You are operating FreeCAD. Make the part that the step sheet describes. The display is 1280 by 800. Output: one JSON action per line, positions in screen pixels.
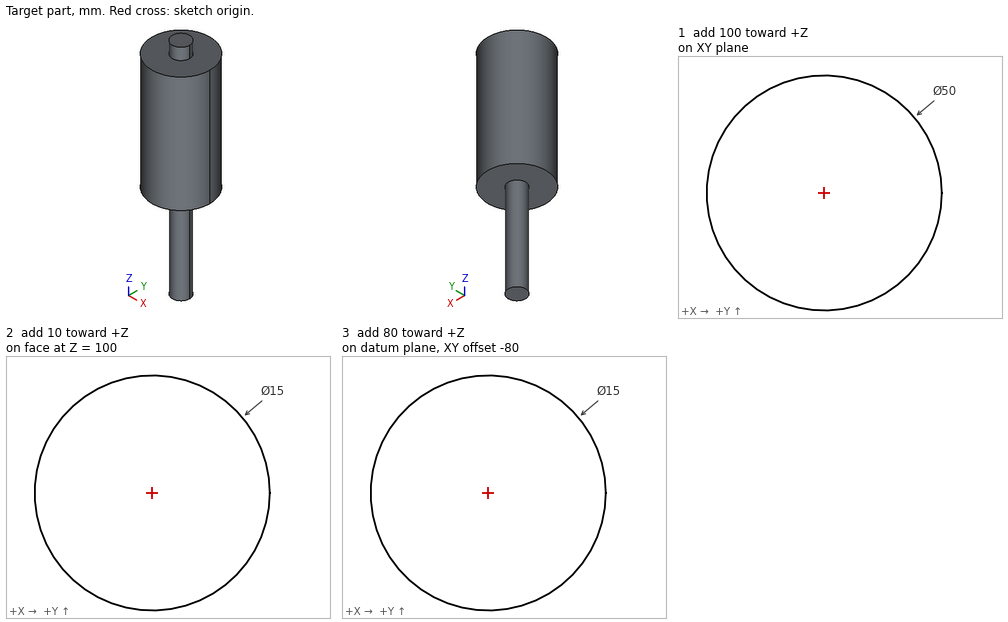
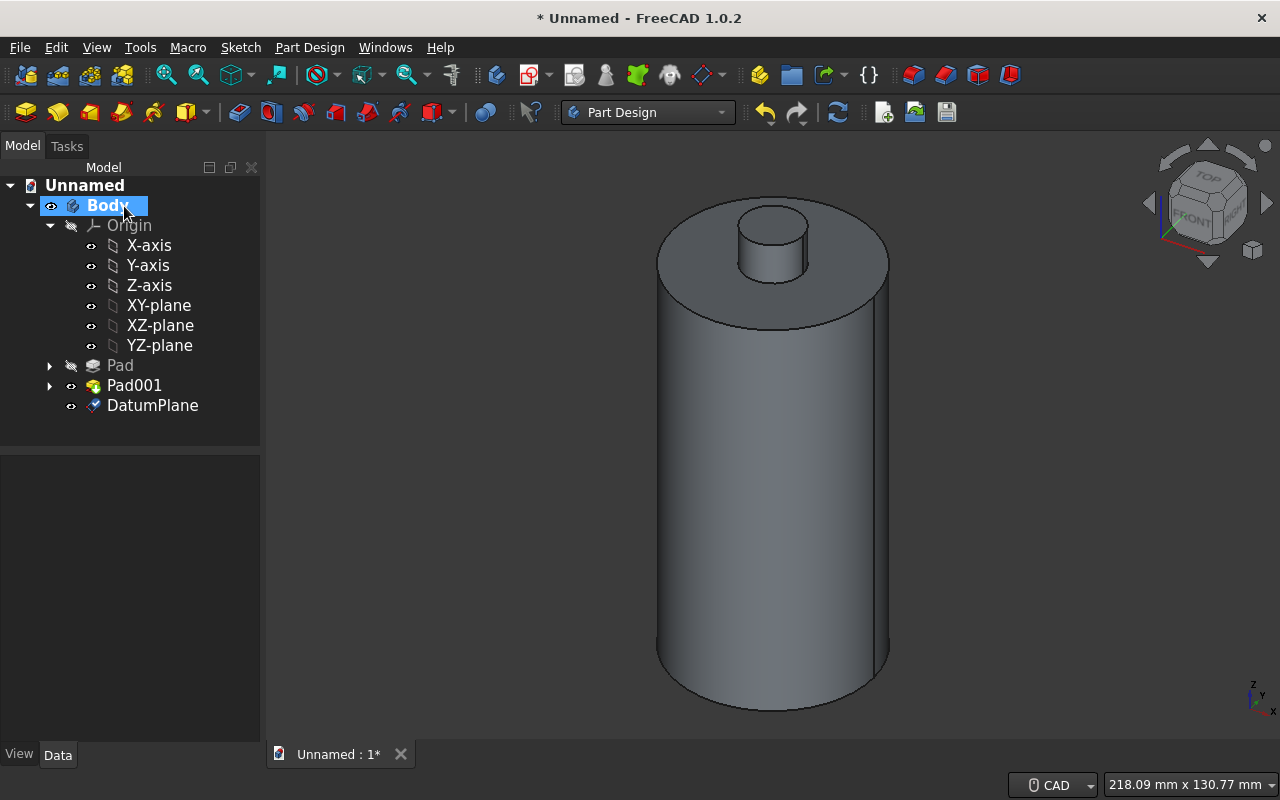
{"action": "left_click", "coordinate": [116, 406]}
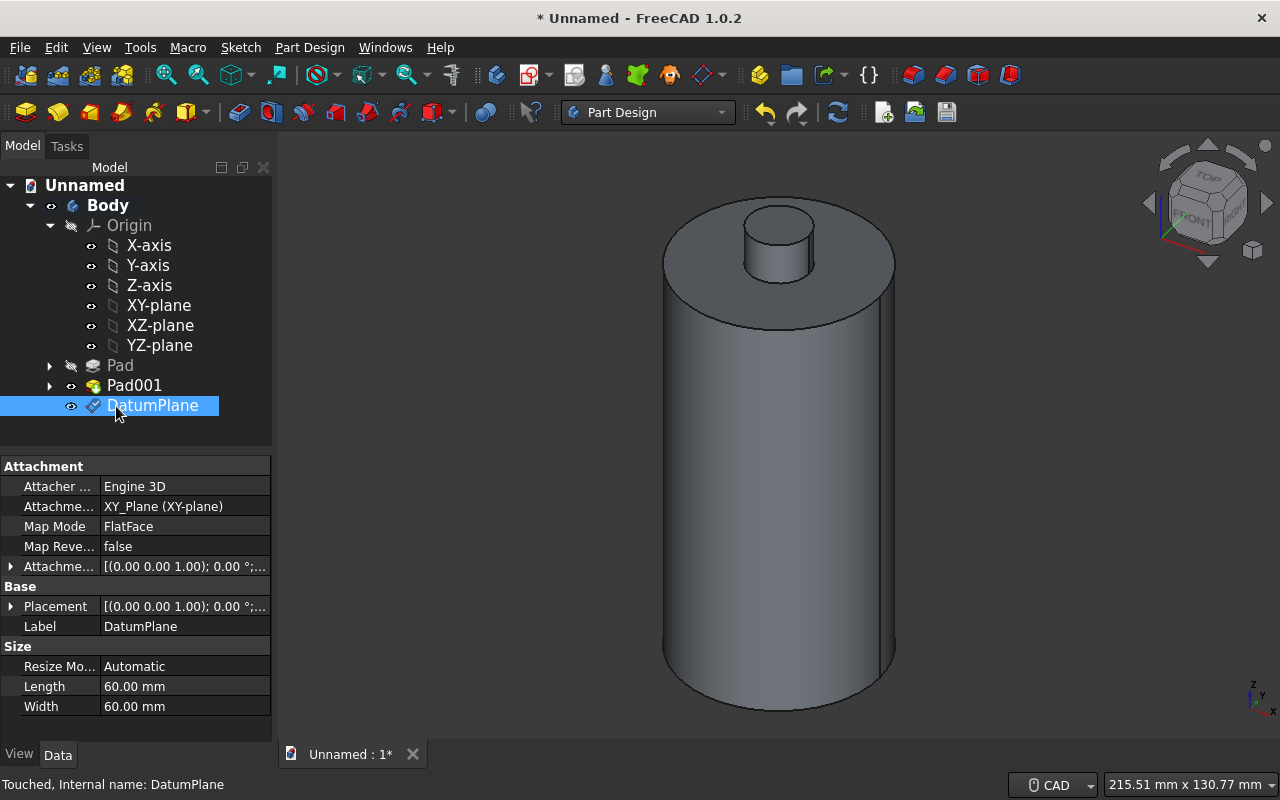
{"action": "left_click", "coordinate": [530, 76]}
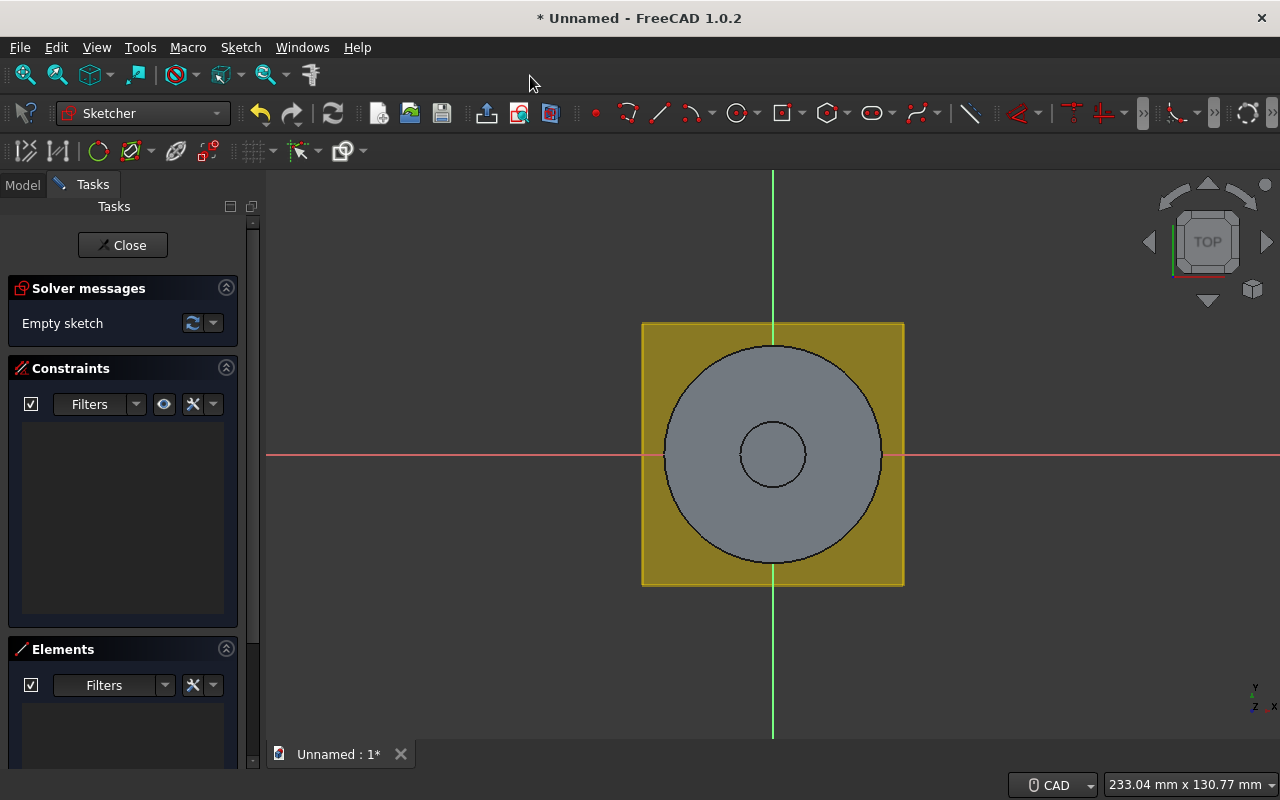
{"action": "left_click", "coordinate": [552, 114]}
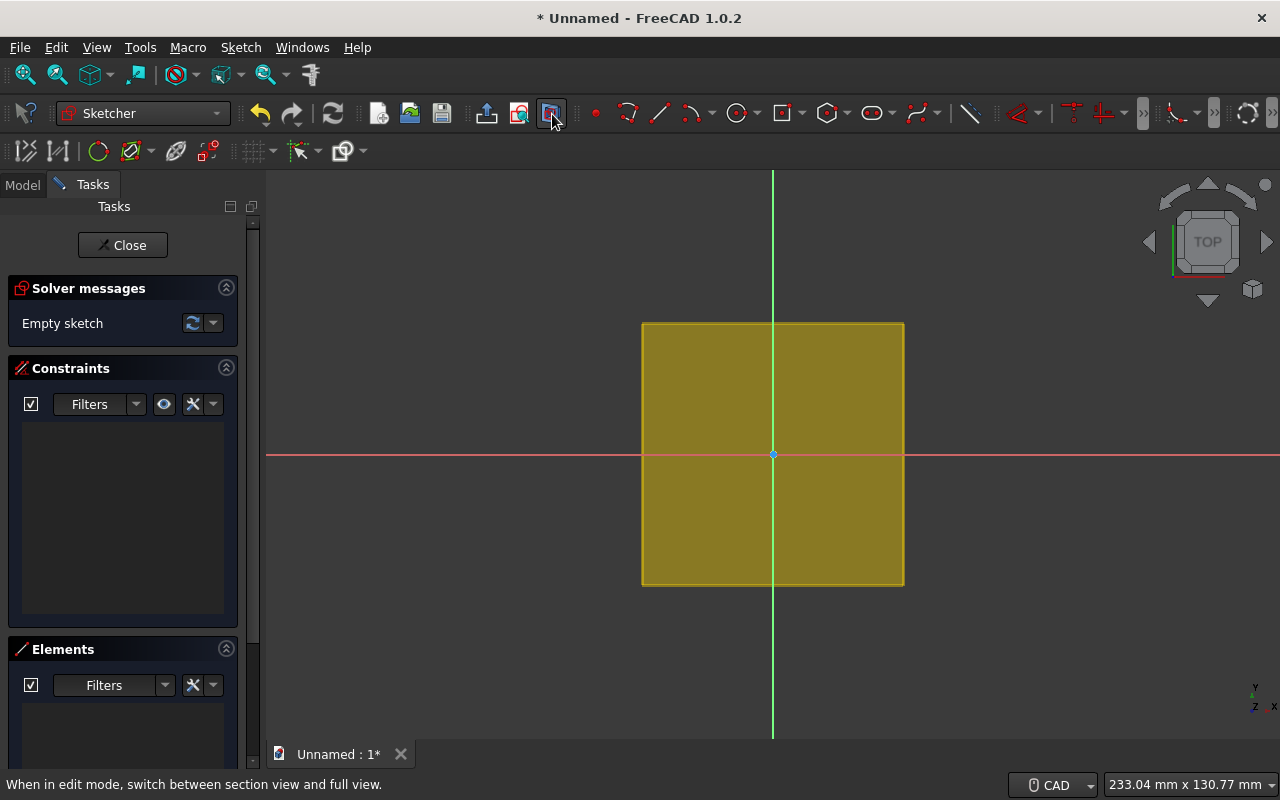
{"action": "scroll", "coordinate": [787, 455], "scroll_direction": "up", "scroll_amount": 9}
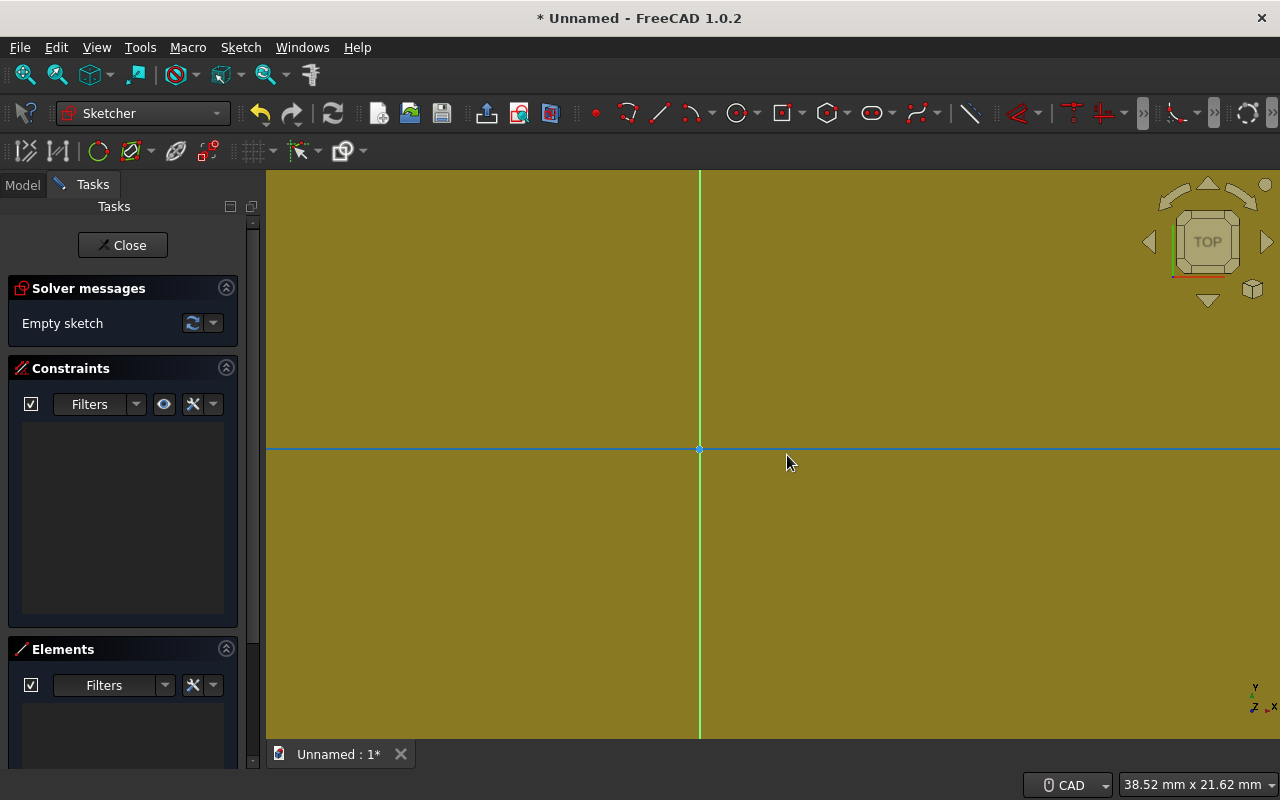
{"action": "left_click", "coordinate": [738, 114]}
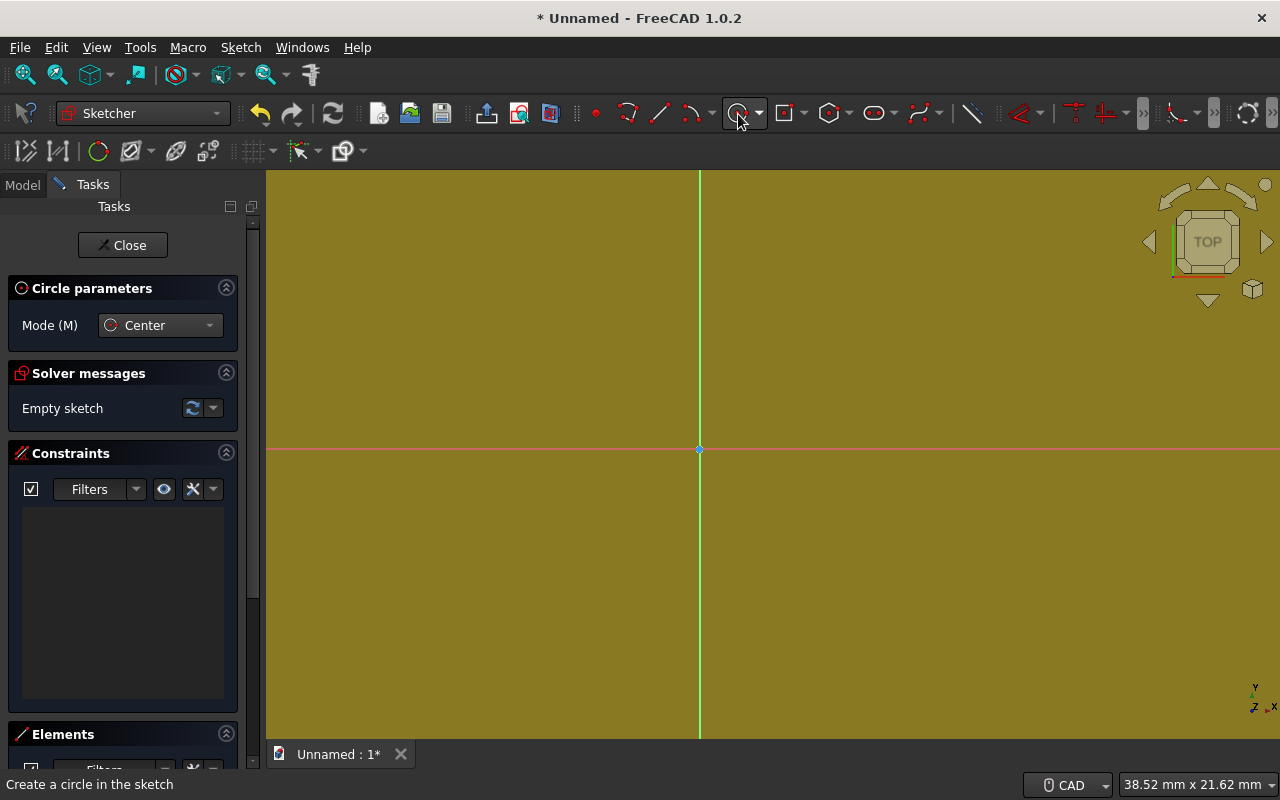
{"action": "left_click", "coordinate": [700, 449]}
{"action": "mouse_move", "coordinate": [839, 310]}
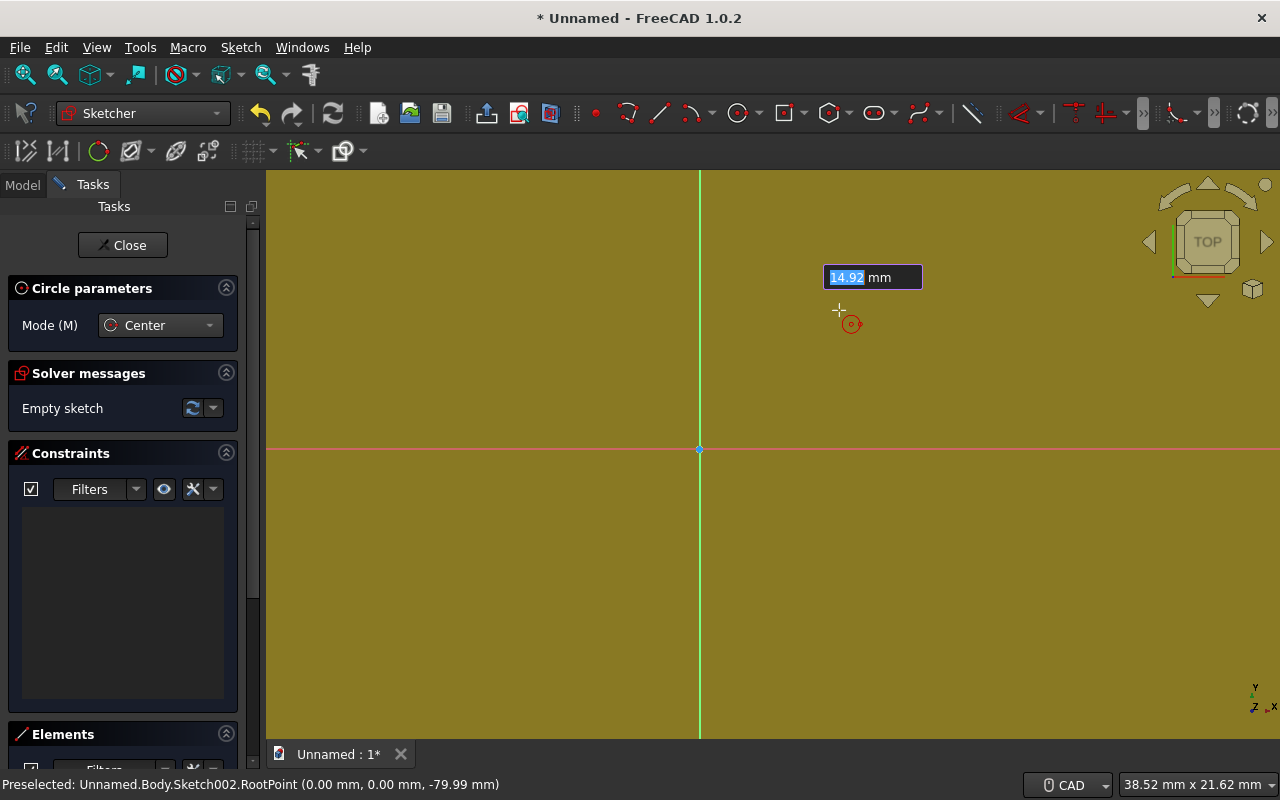
{"action": "type", "text": "15"}
{"action": "key", "text": "Return"}
{"action": "key", "text": "Escape"}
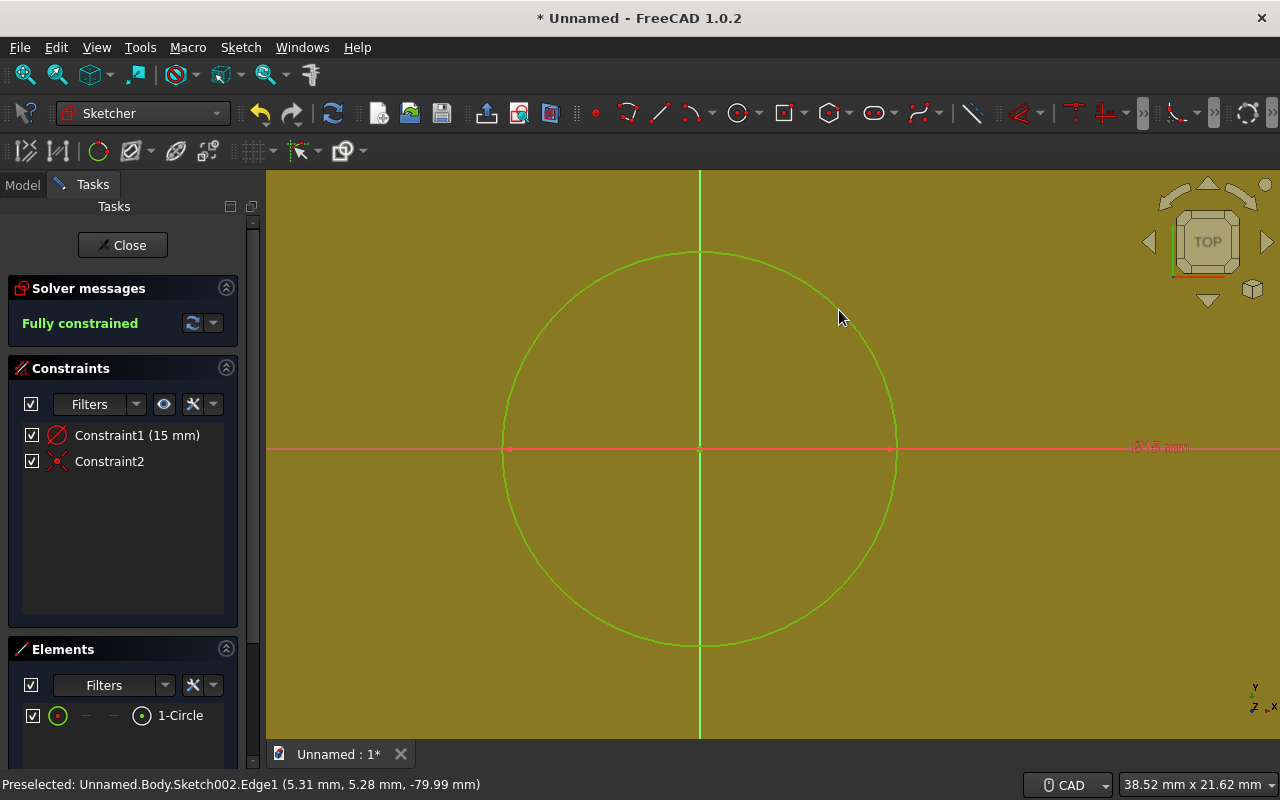
{"action": "left_click", "coordinate": [123, 245]}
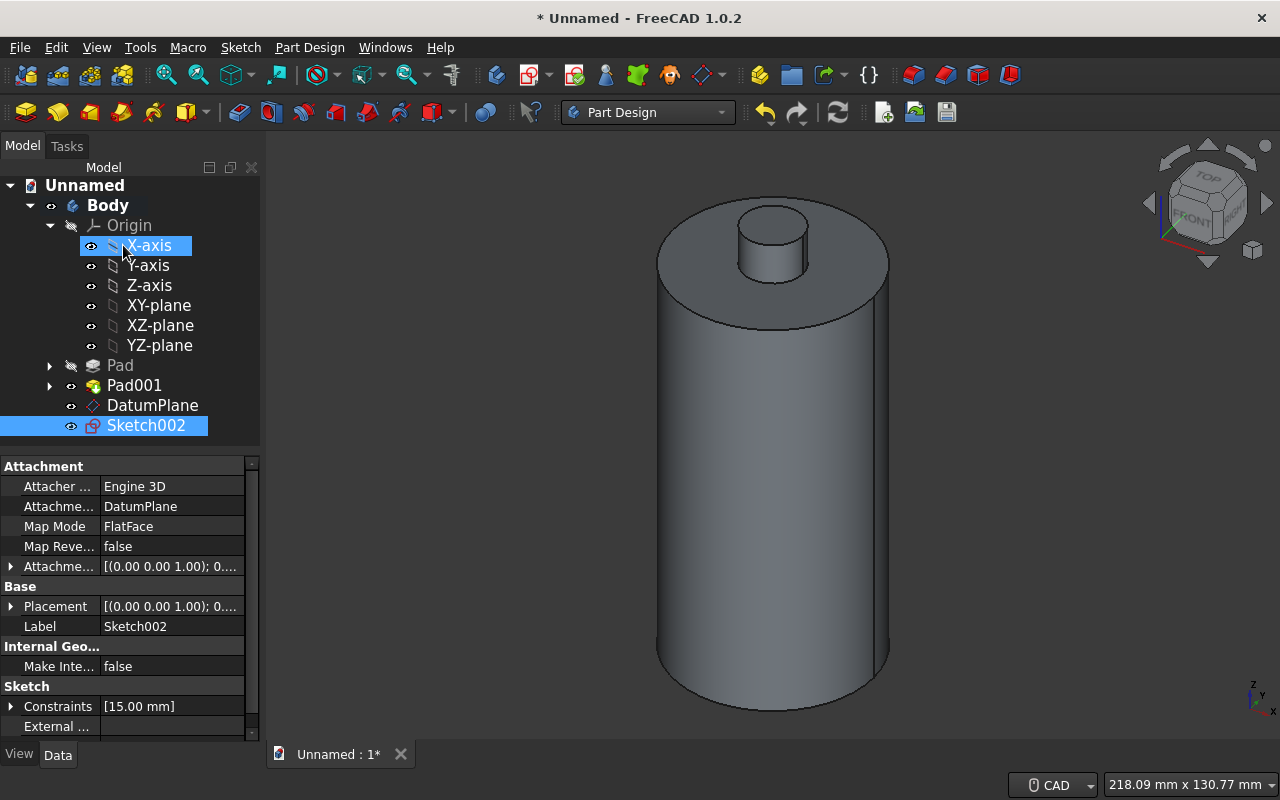
{"action": "left_click", "coordinate": [26, 112]}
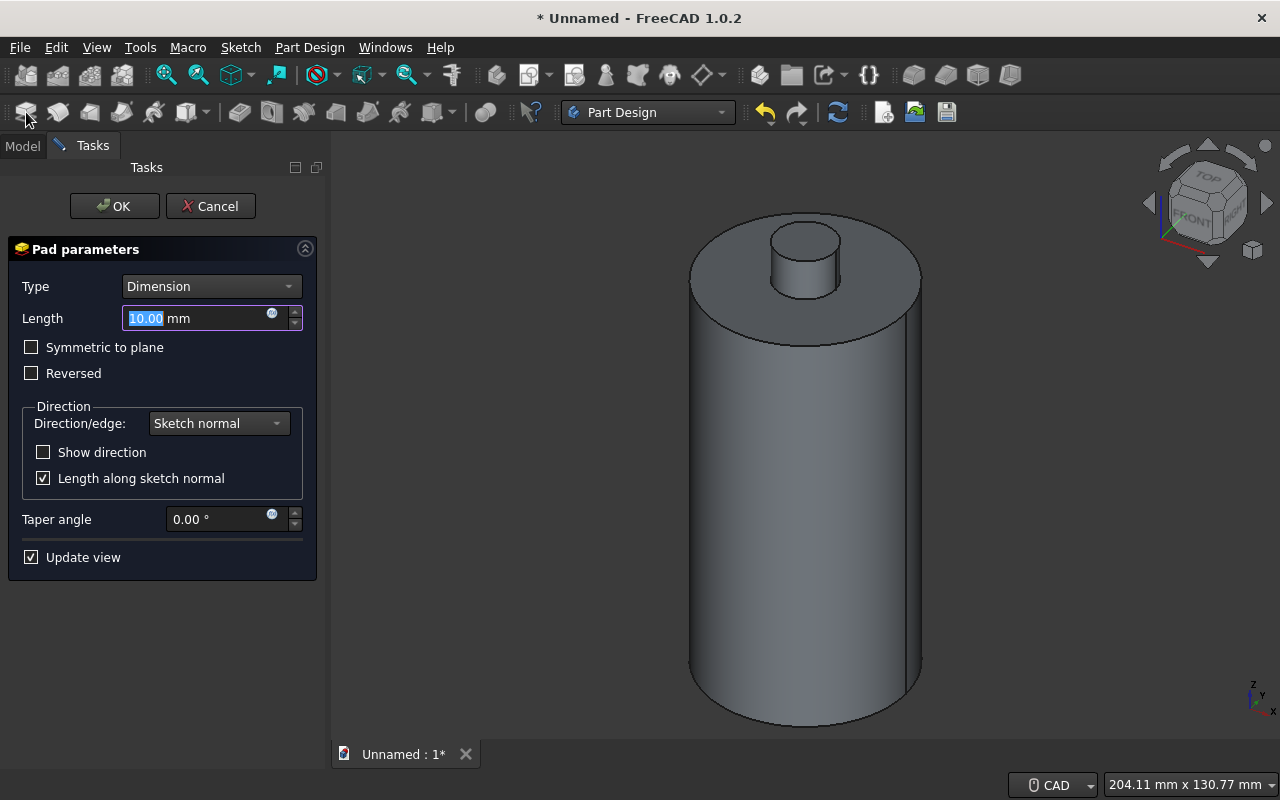
{"action": "type", "text": "80"}
{"action": "key", "text": "Tab"}